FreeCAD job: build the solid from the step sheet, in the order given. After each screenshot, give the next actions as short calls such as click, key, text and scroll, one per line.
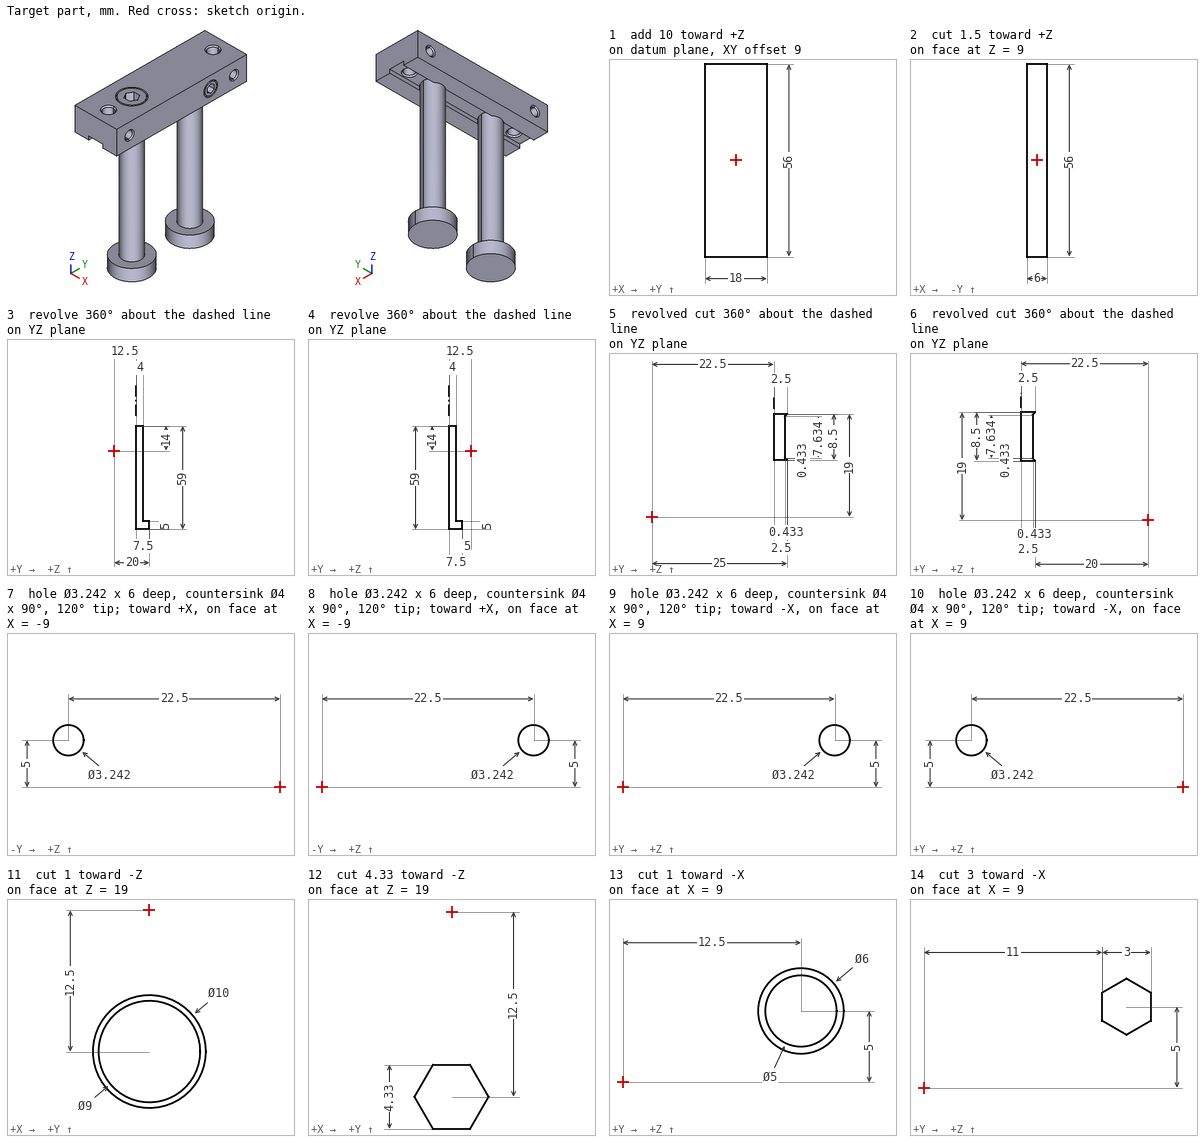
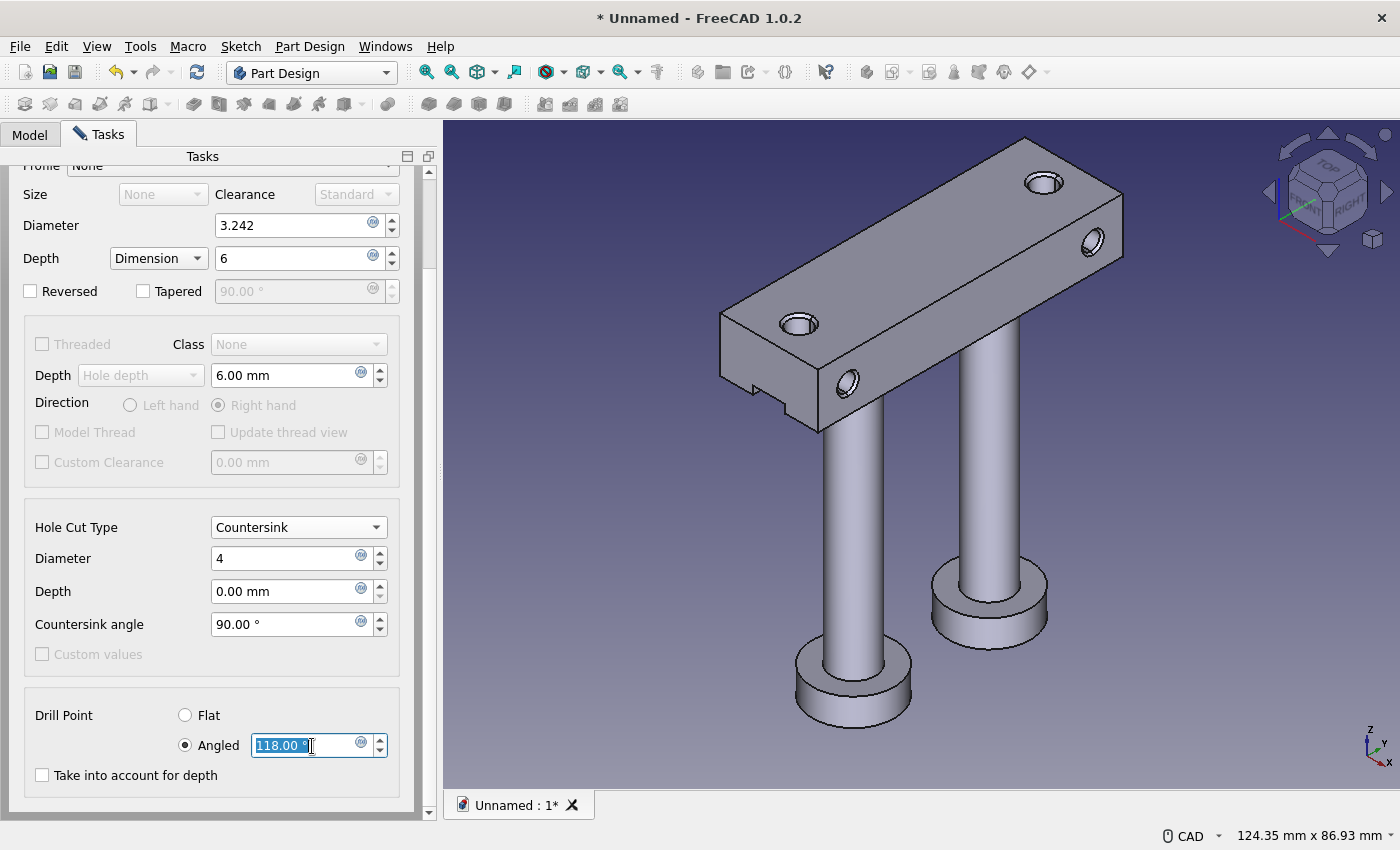
text(120)
key(Tab)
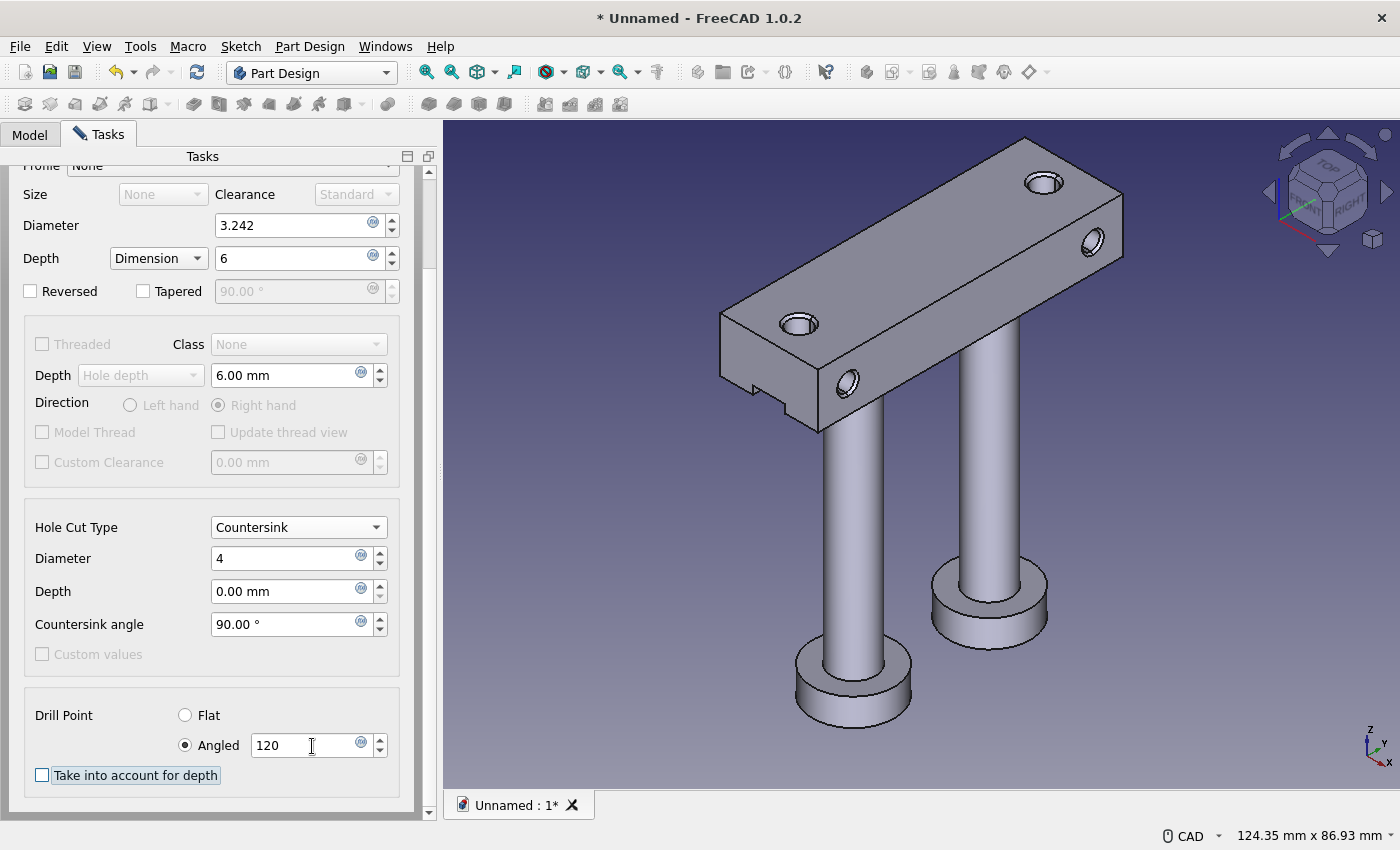
scroll(429, 493, up, 3)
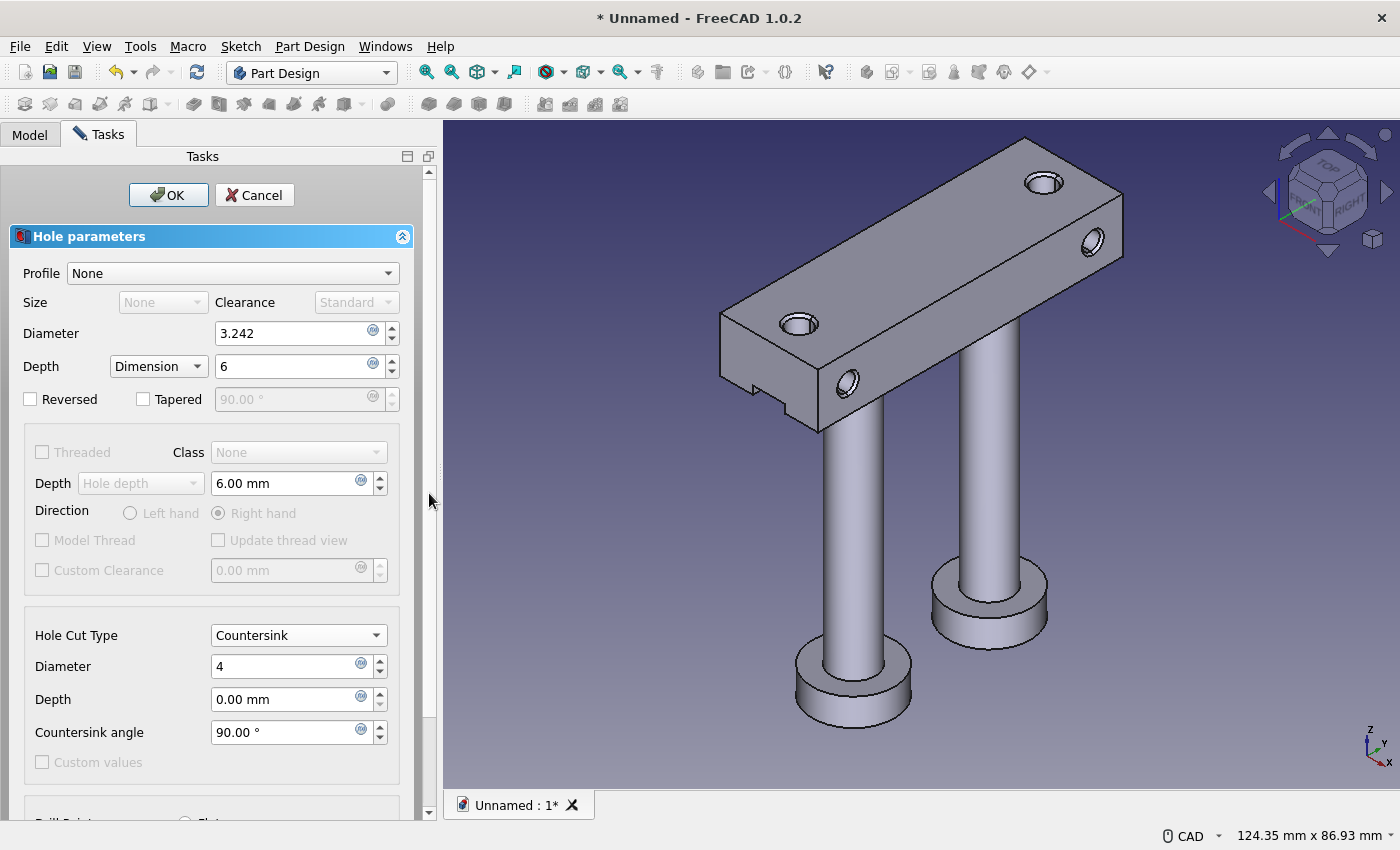
click(169, 195)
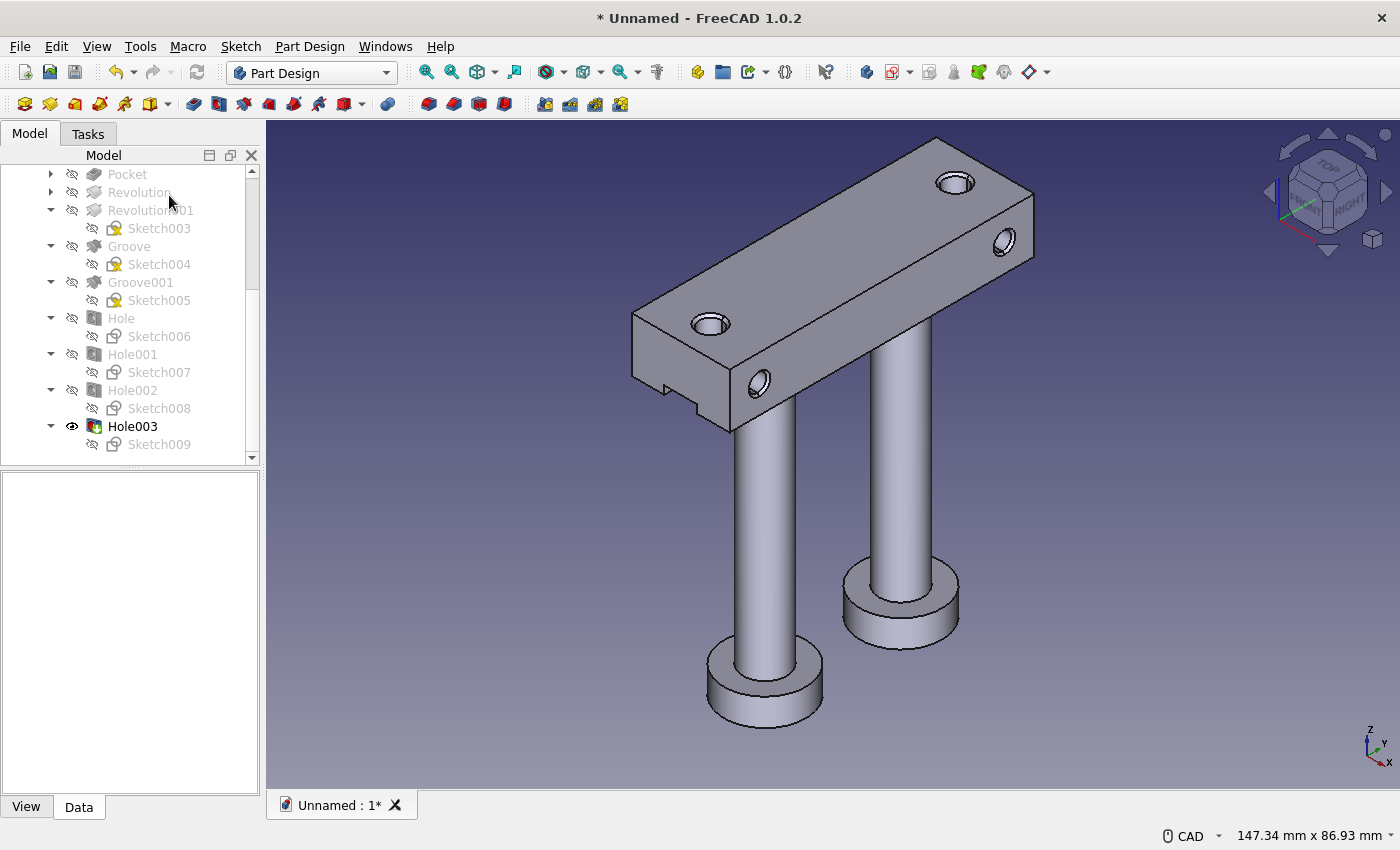
click(877, 227)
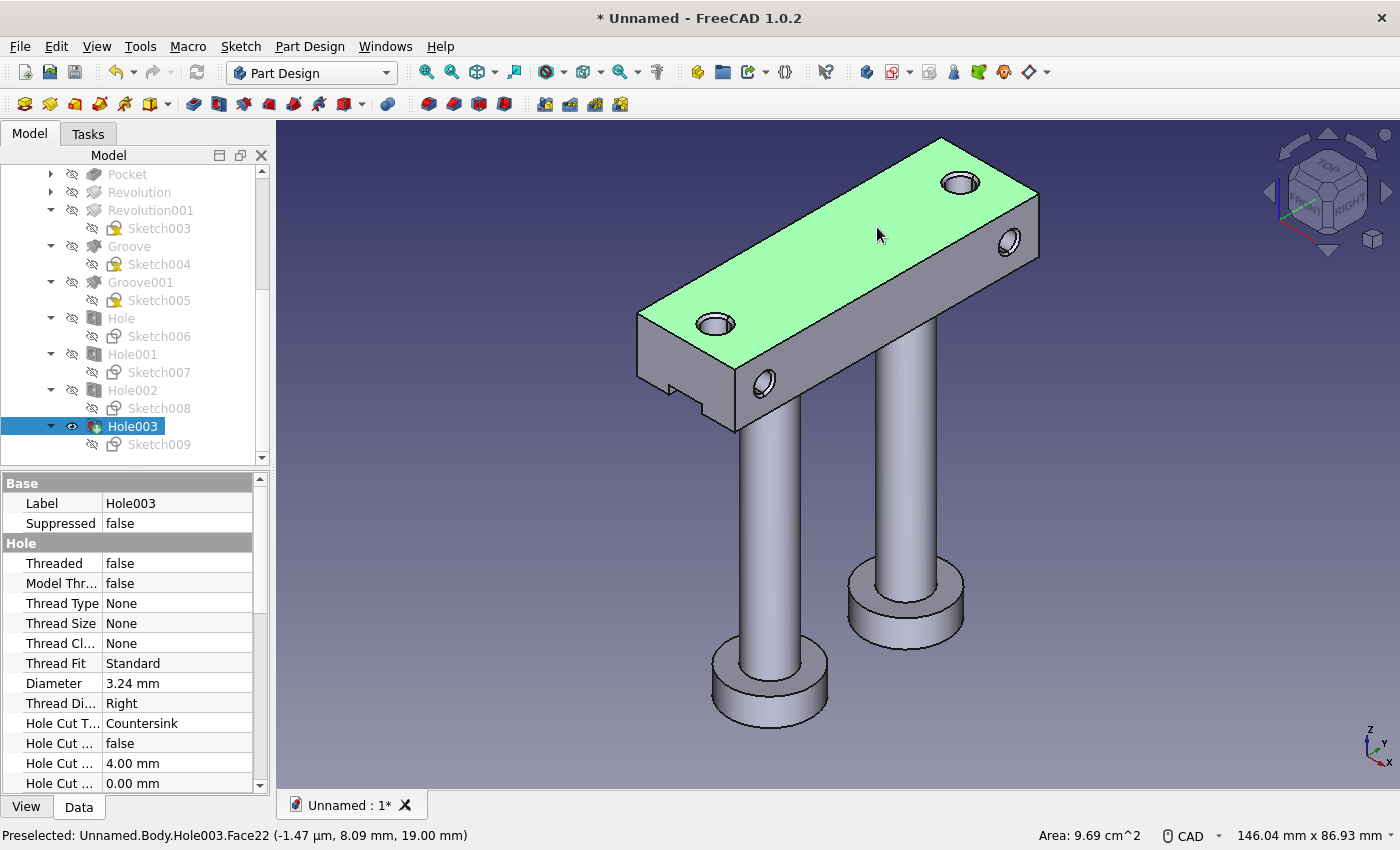
click(892, 72)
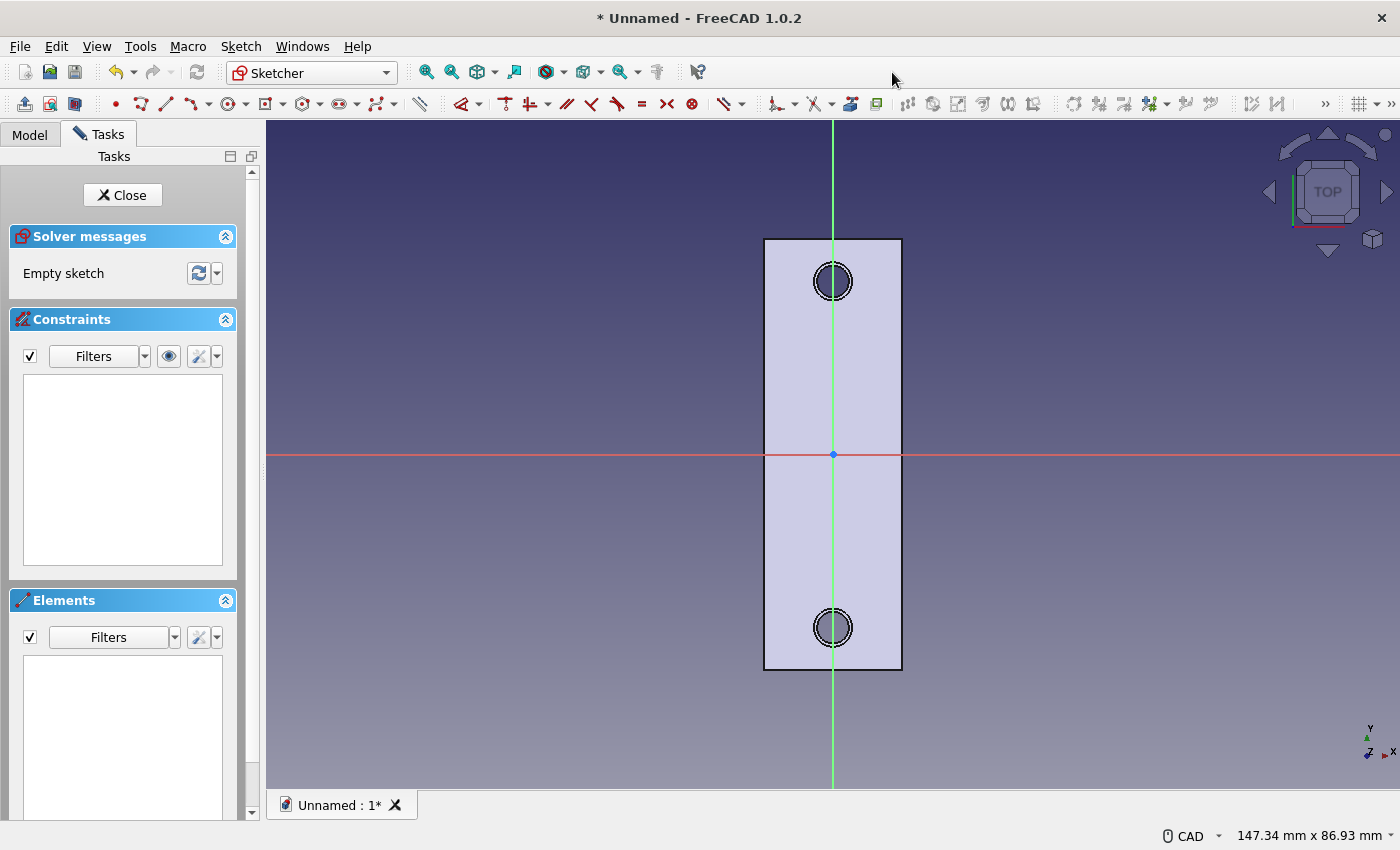
scroll(863, 551, up, 6)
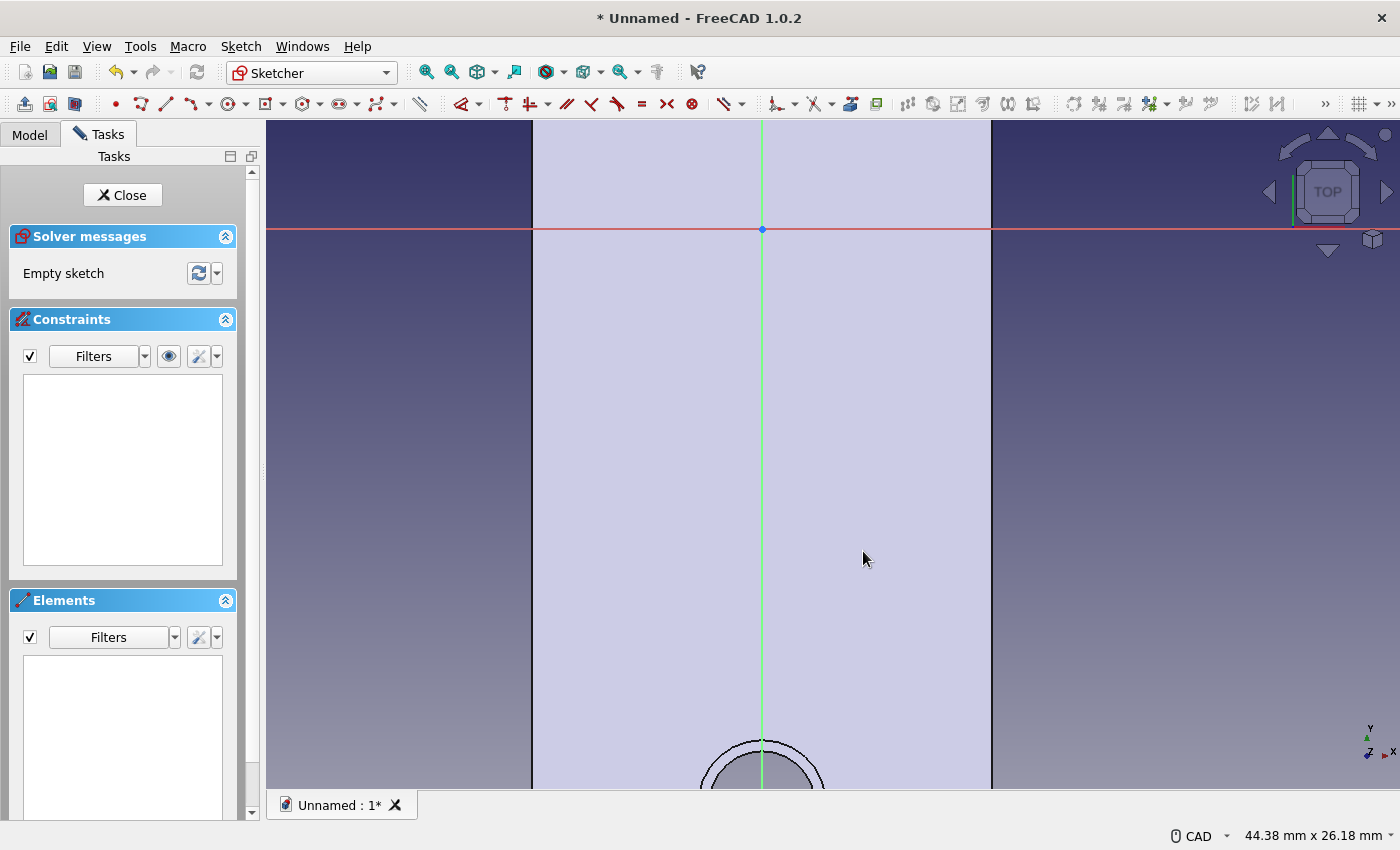
click(228, 104)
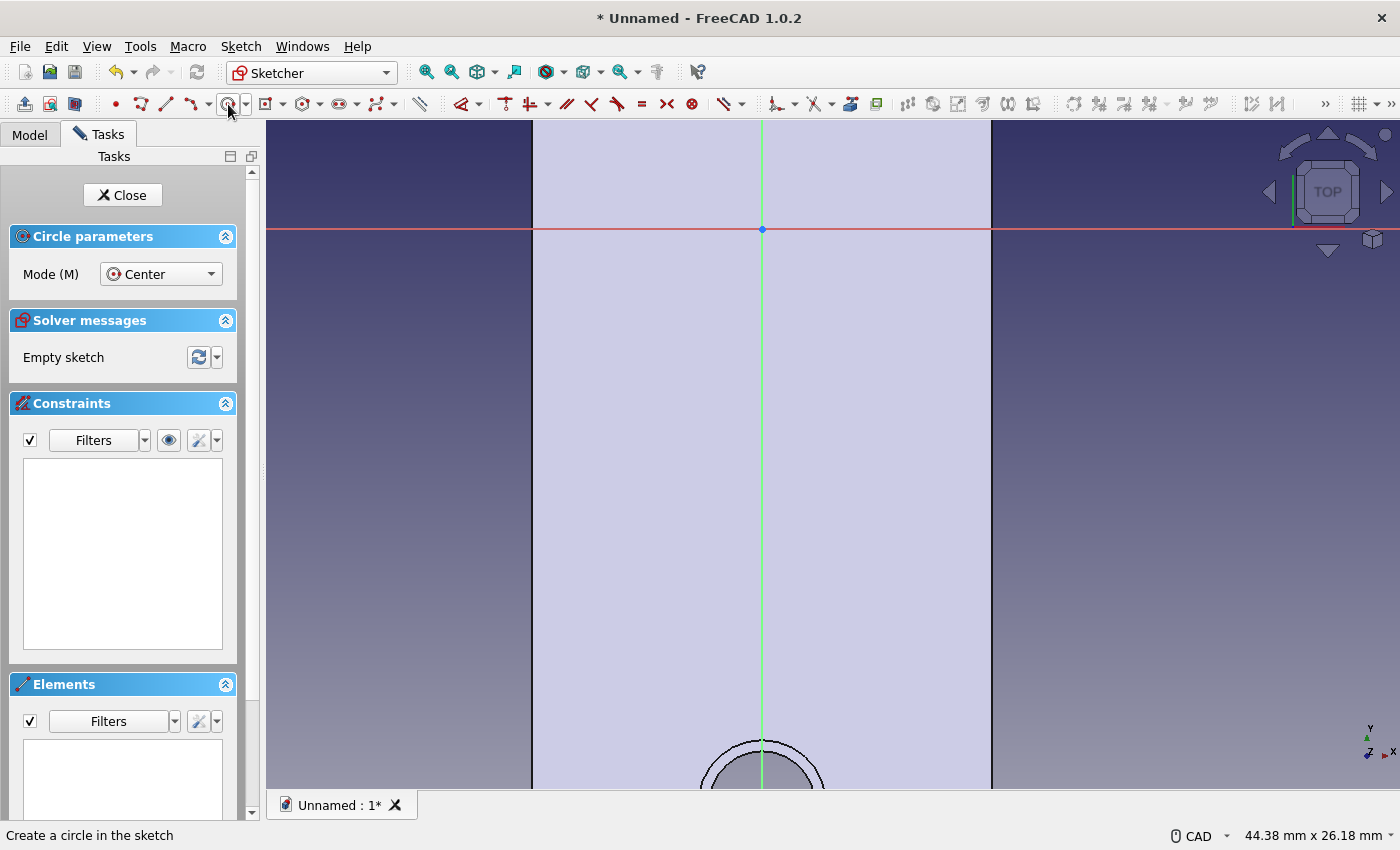
click(762, 549)
move(853, 458)